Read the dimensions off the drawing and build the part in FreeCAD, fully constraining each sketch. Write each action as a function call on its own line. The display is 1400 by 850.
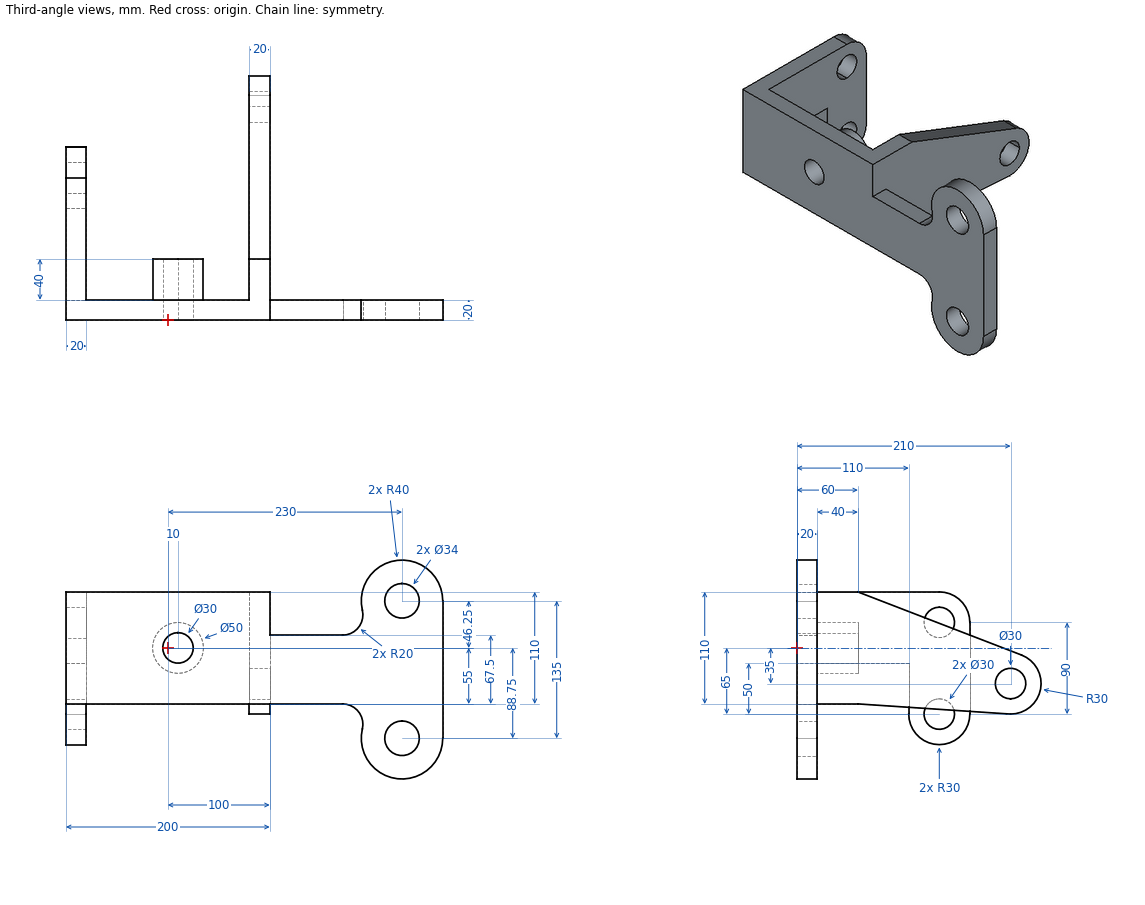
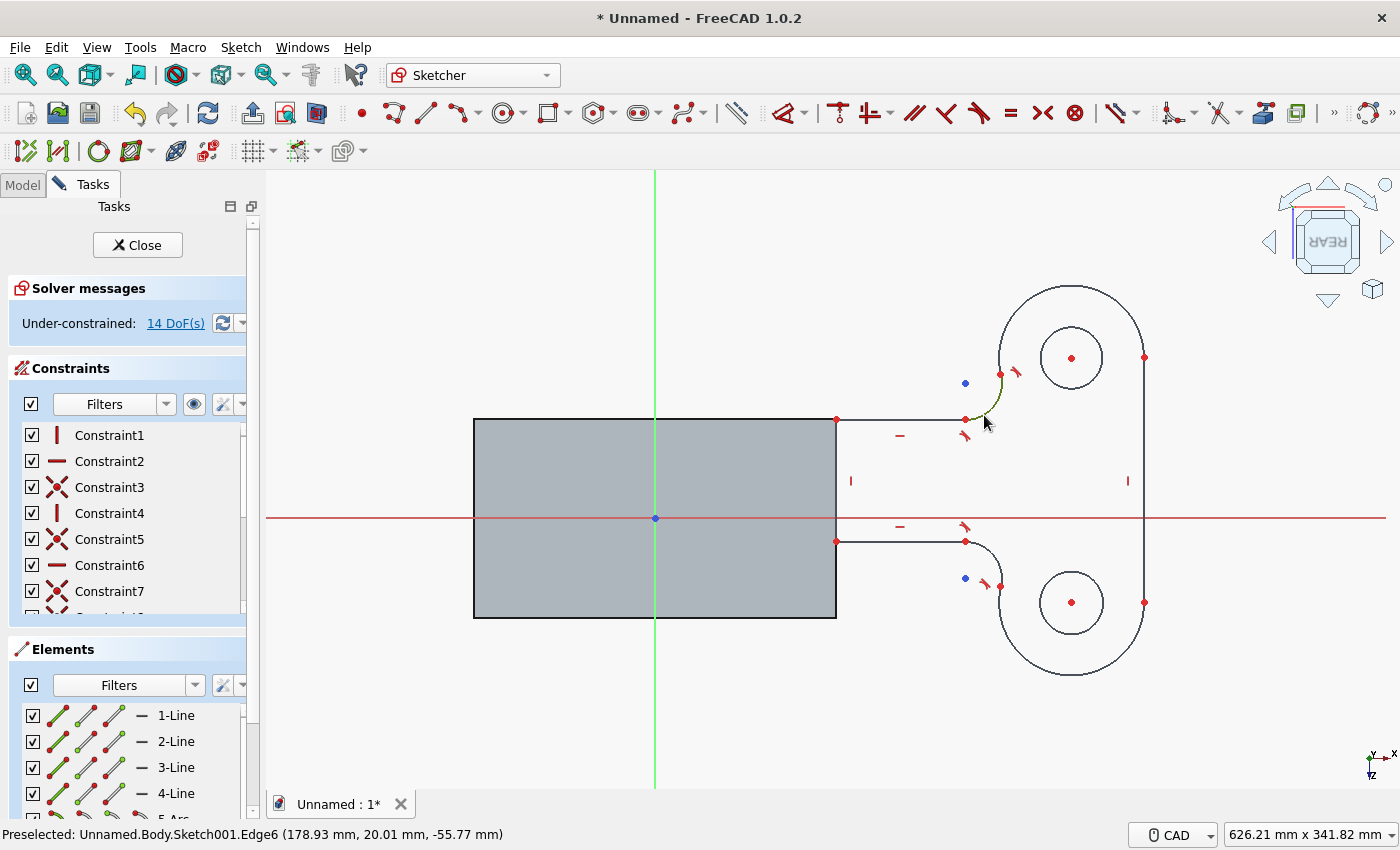
click(1000, 567)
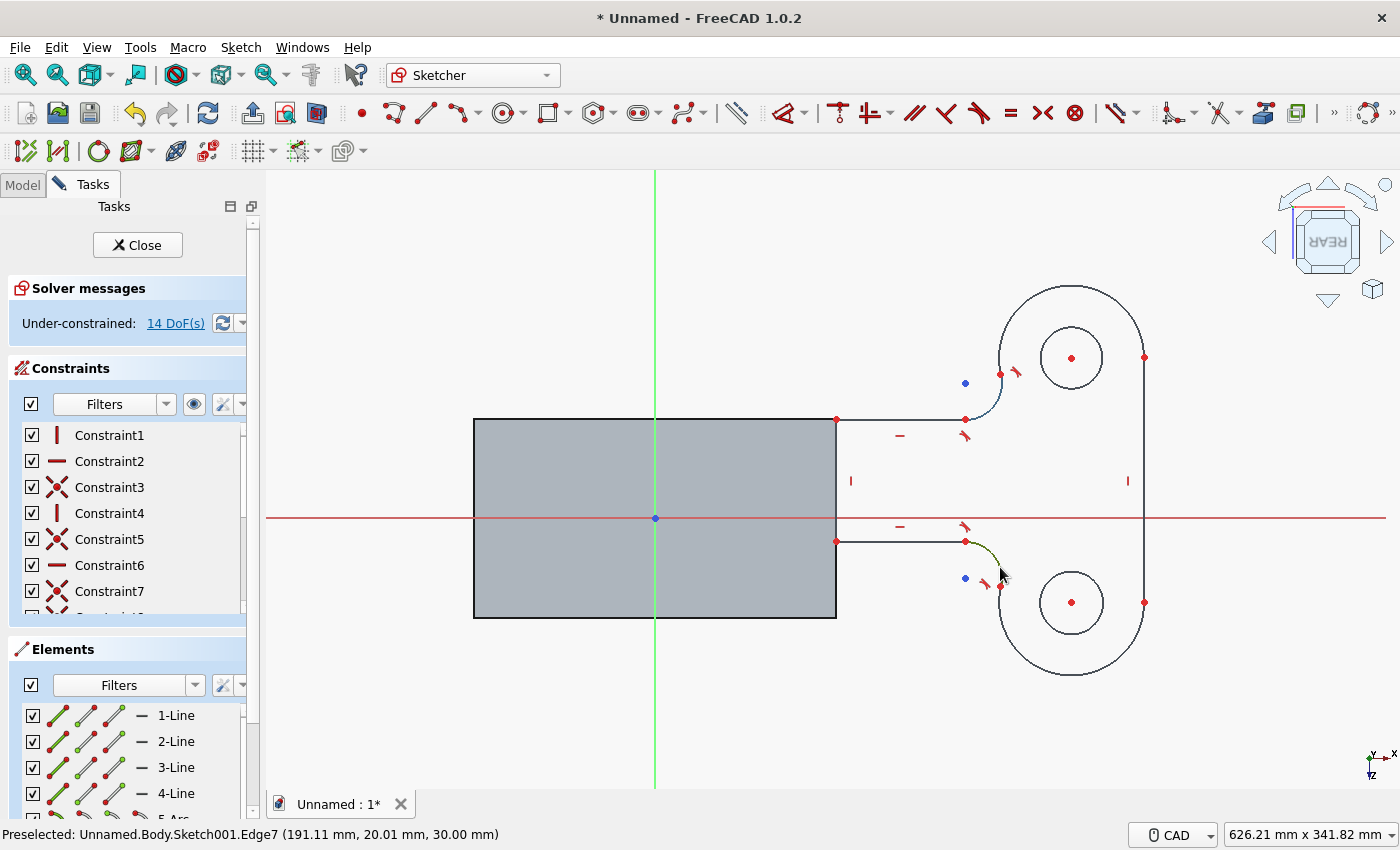
key(e)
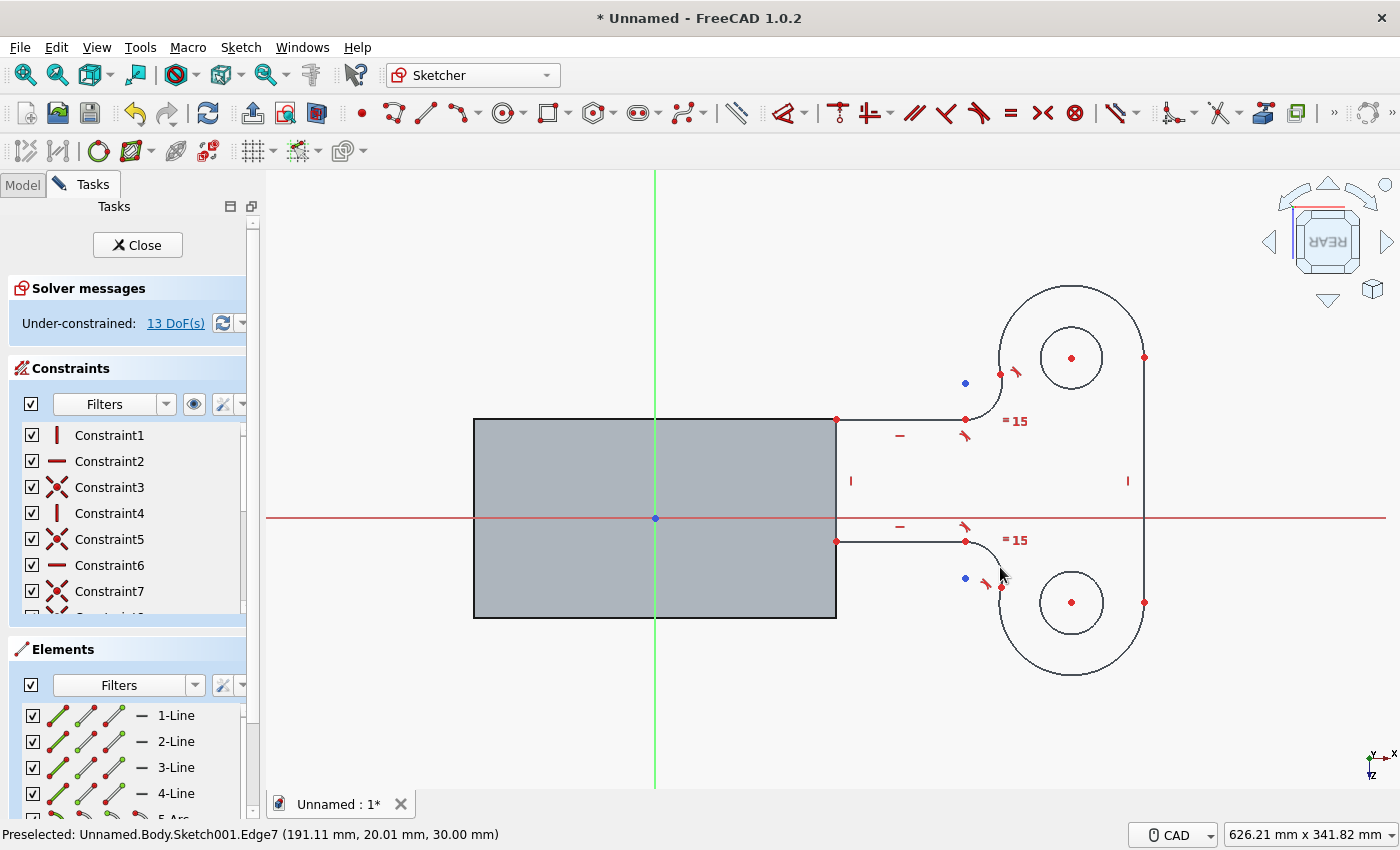
click(1110, 297)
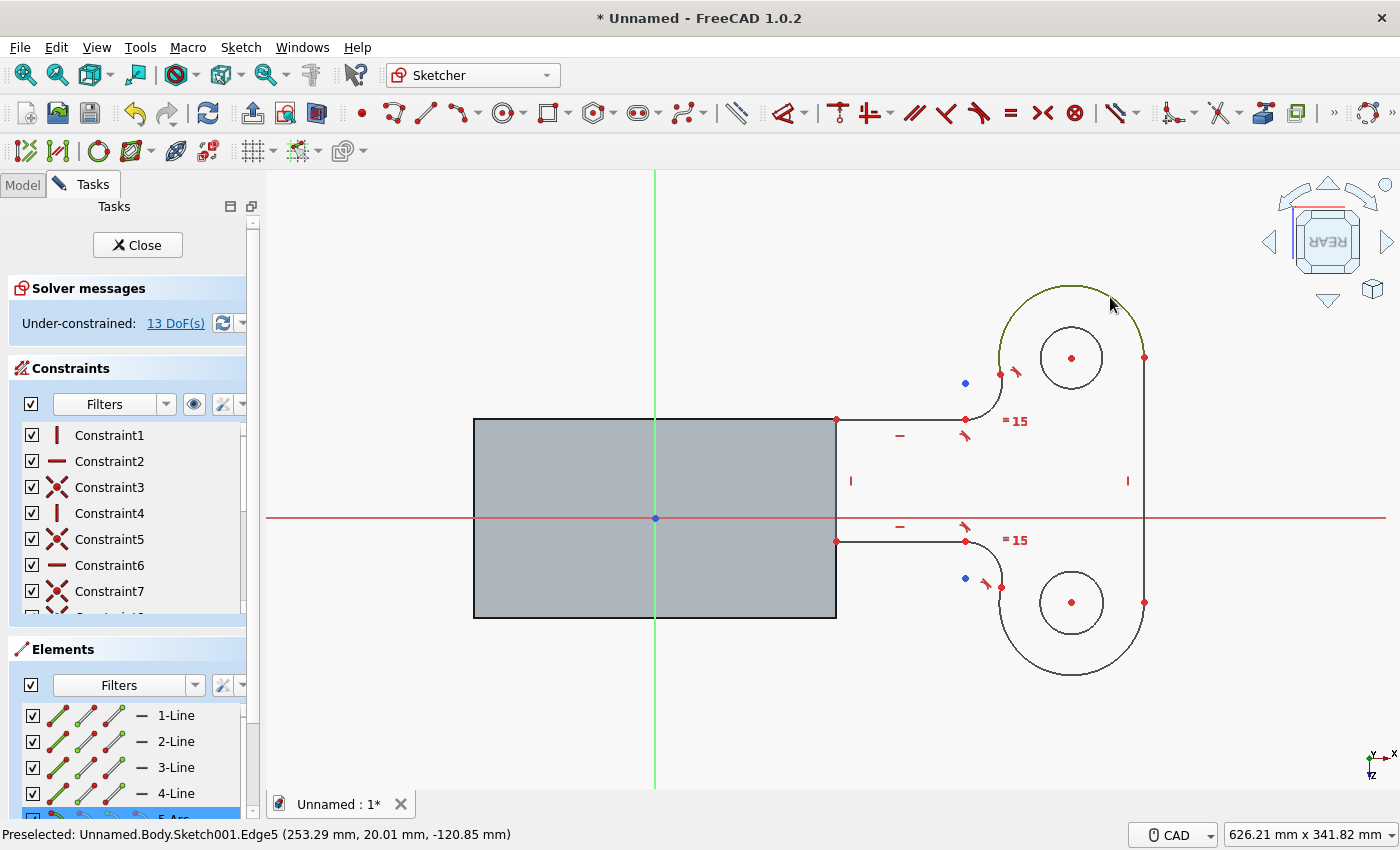
click(1021, 654)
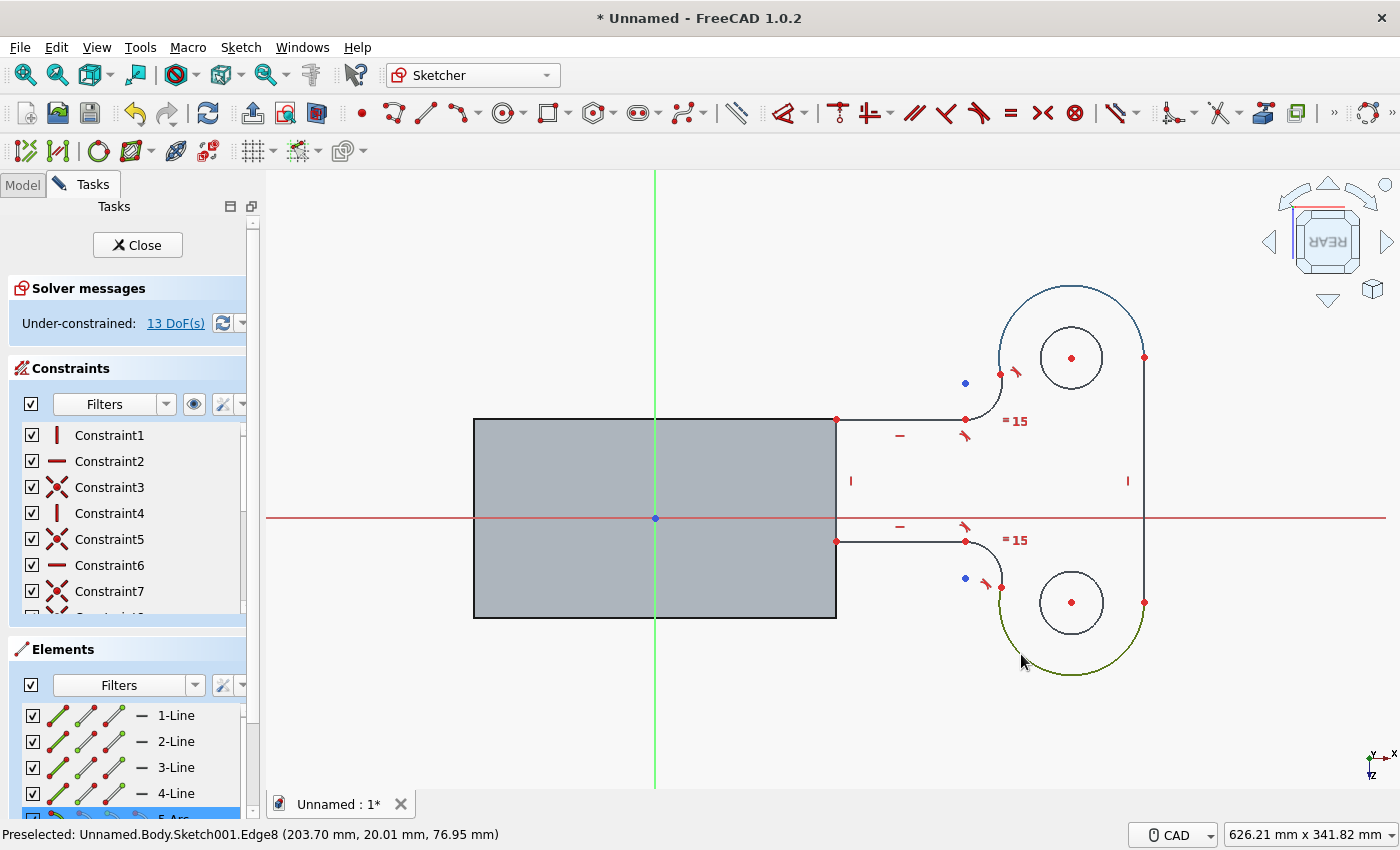
key(e)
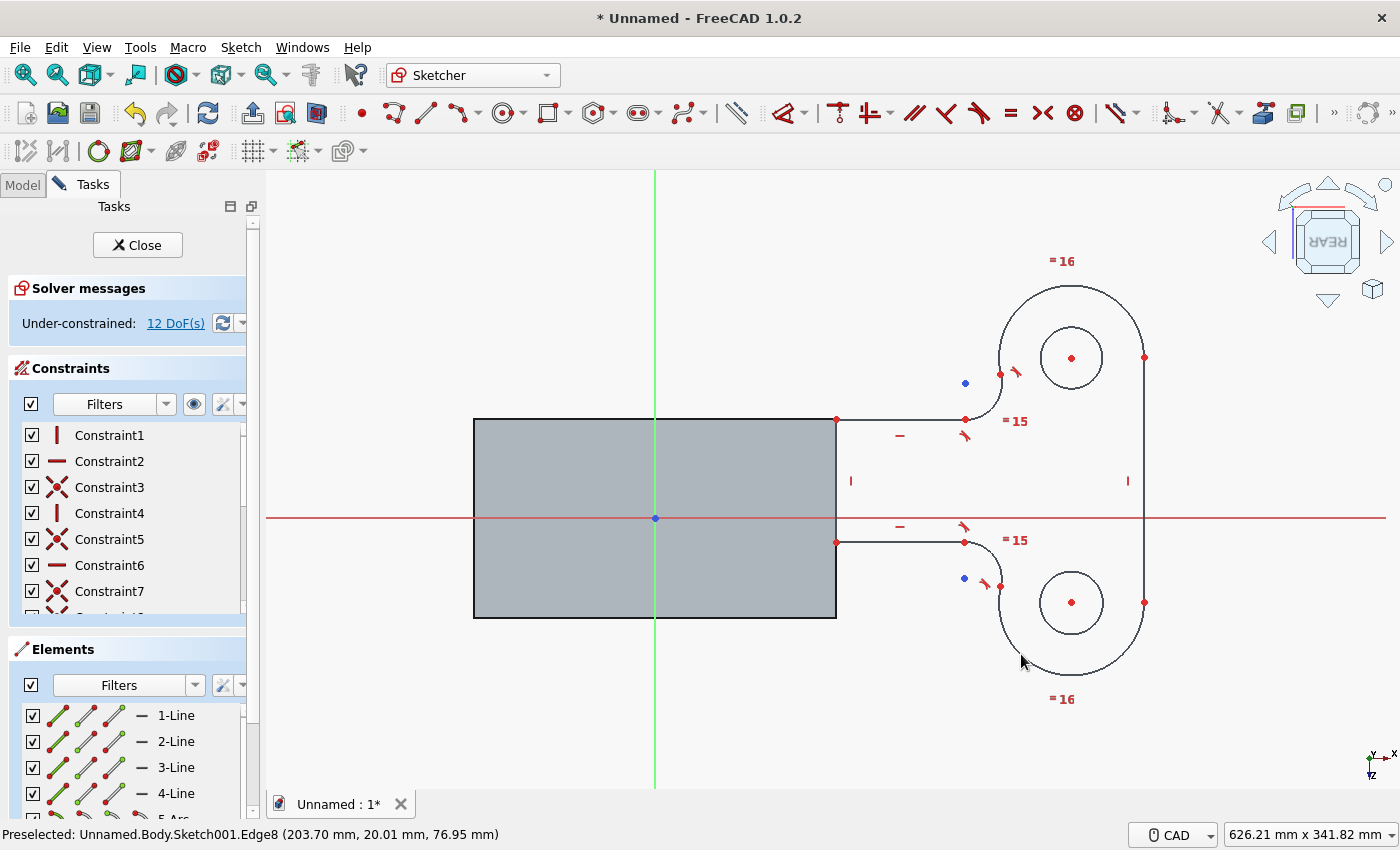
click(1094, 581)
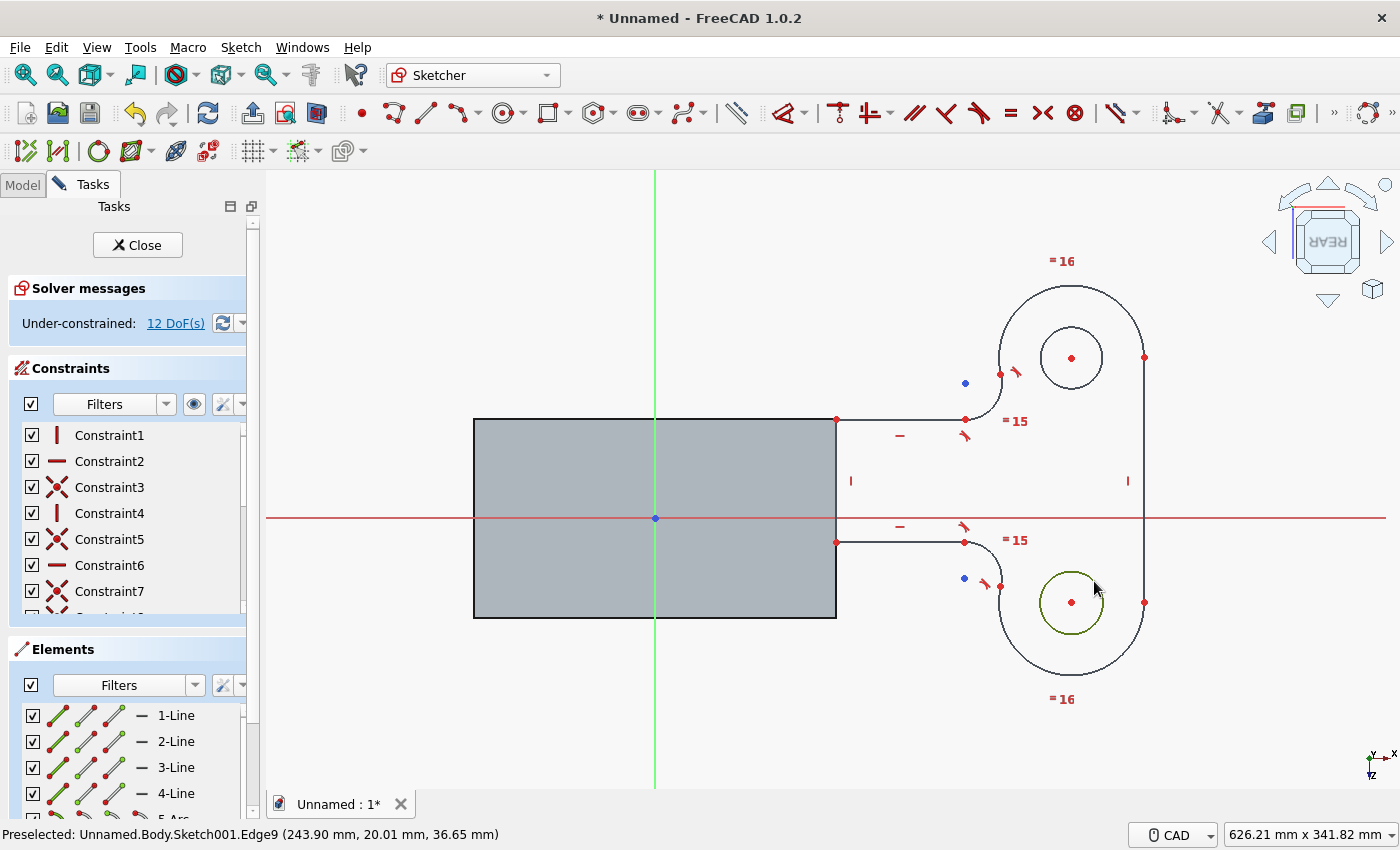
click(1093, 336)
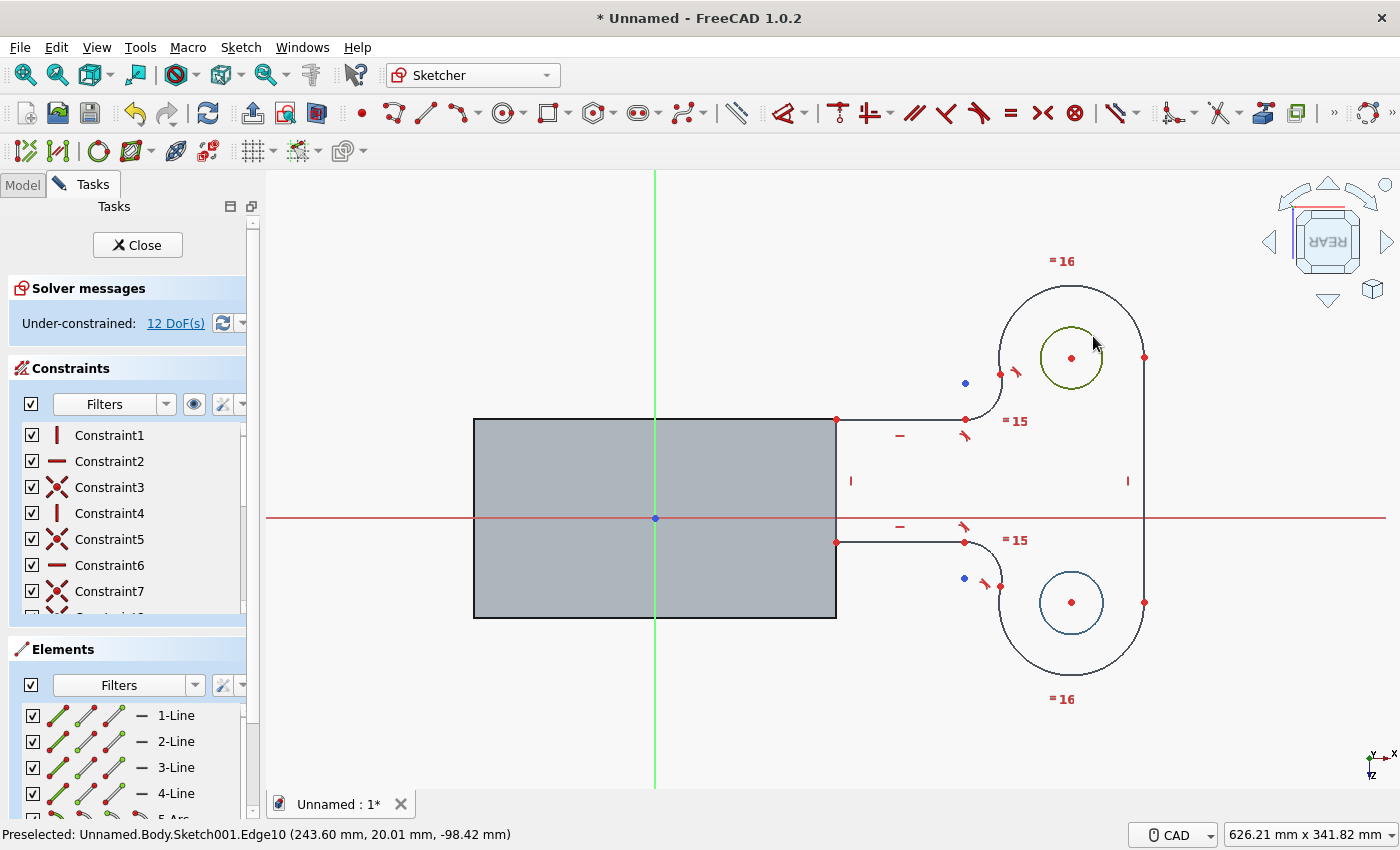
click(1012, 114)